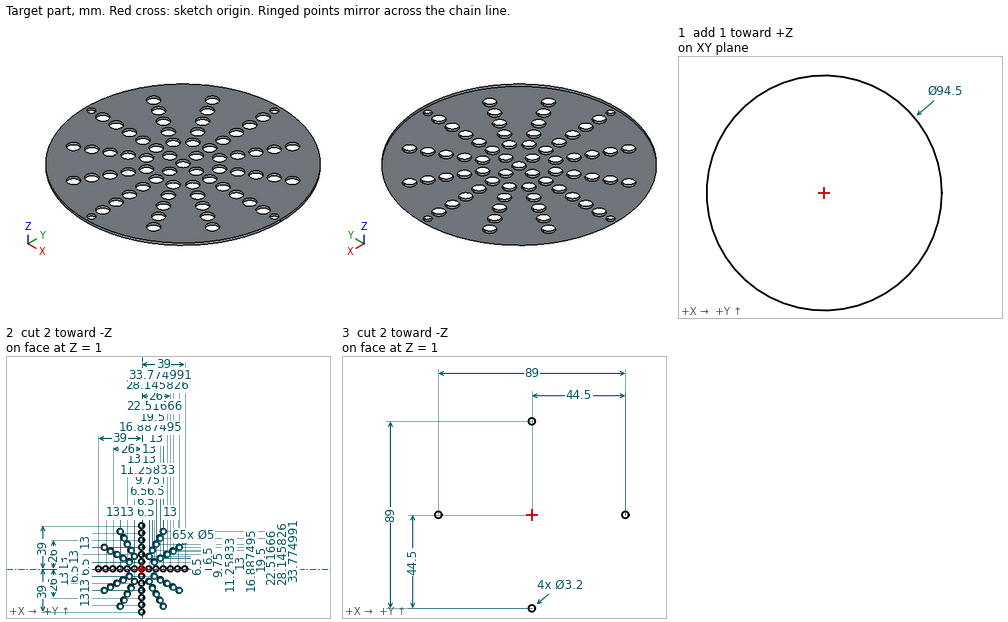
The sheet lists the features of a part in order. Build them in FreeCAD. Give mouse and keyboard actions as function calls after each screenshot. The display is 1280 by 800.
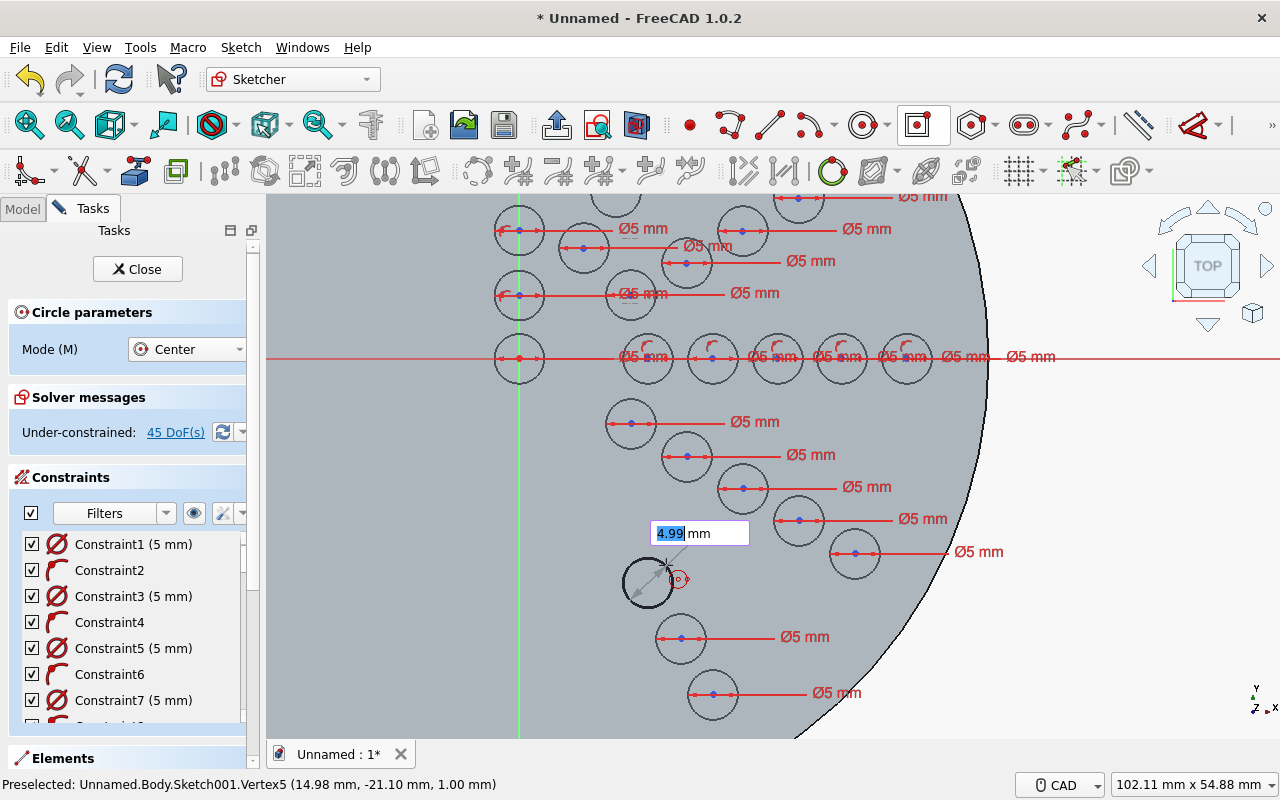
text(5)
key(Return)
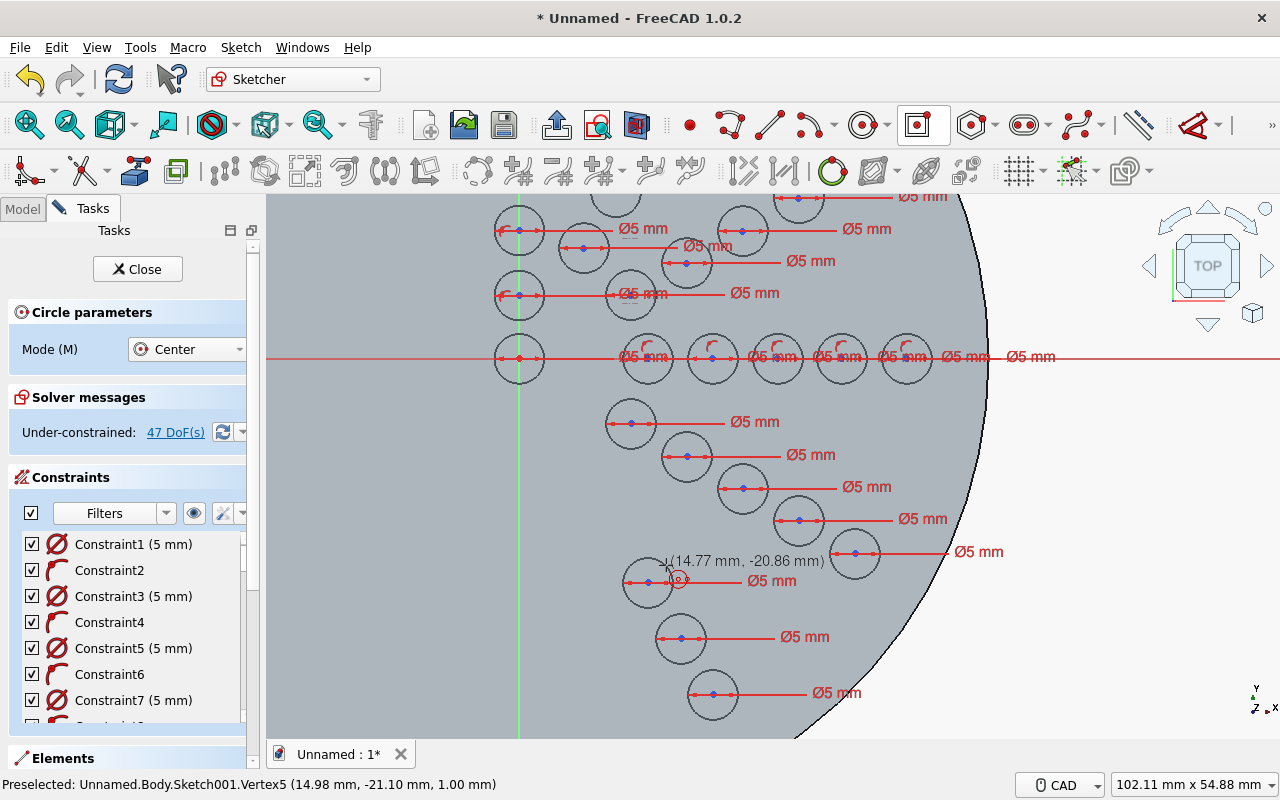
click(616, 527)
move(634, 509)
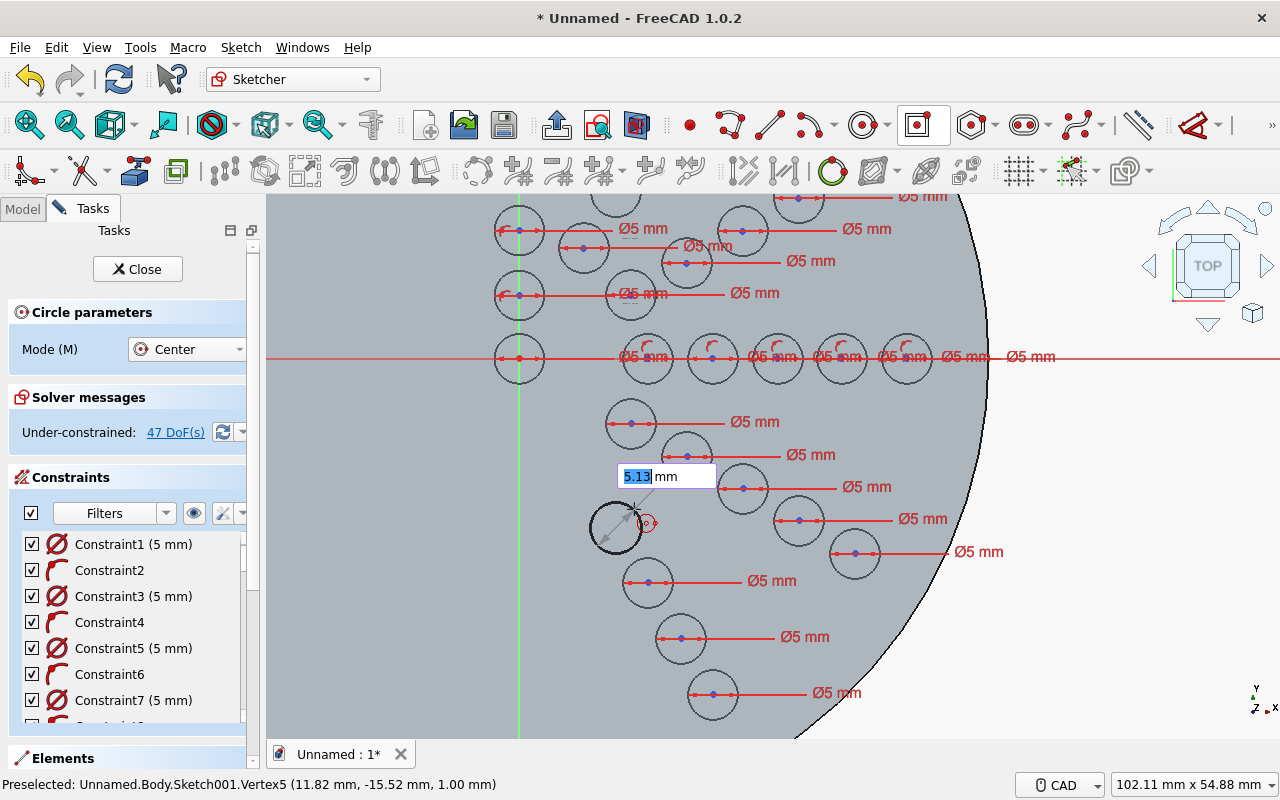
text(5)
key(Return)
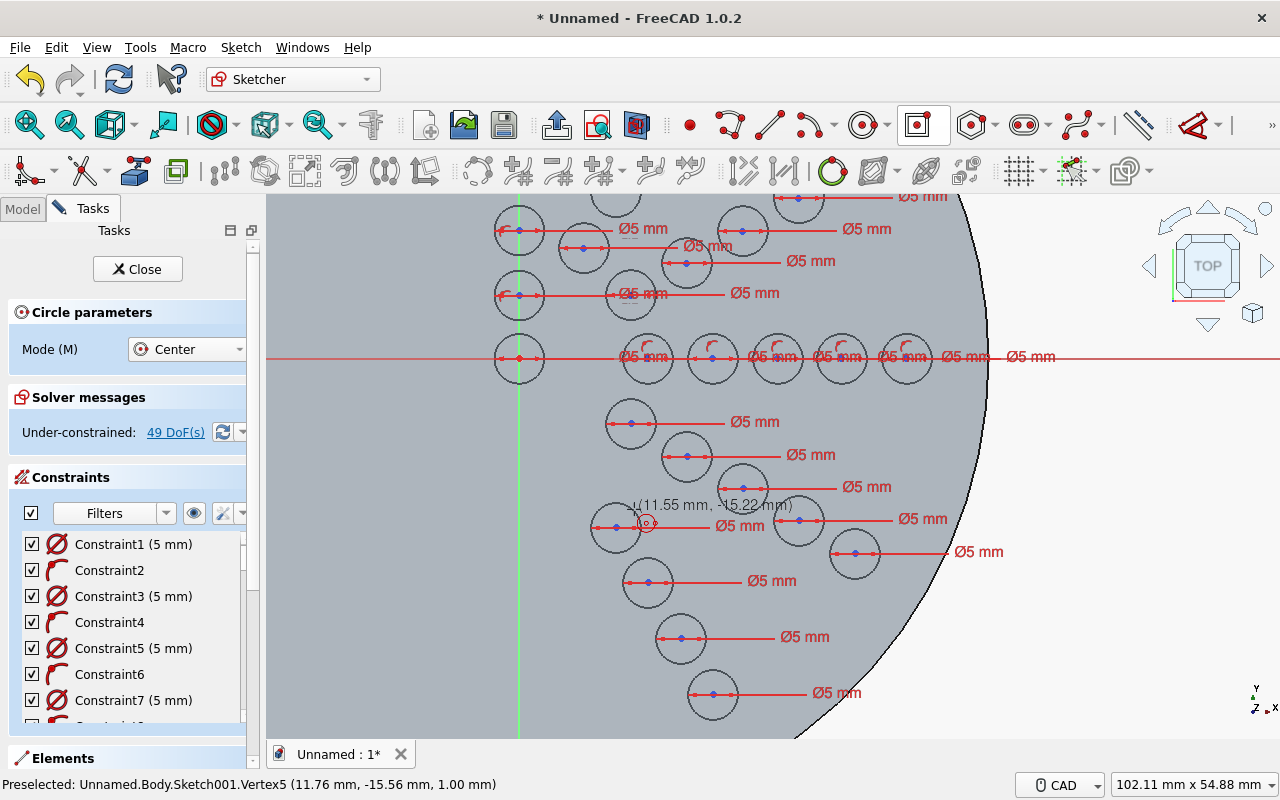
click(584, 471)
move(601, 453)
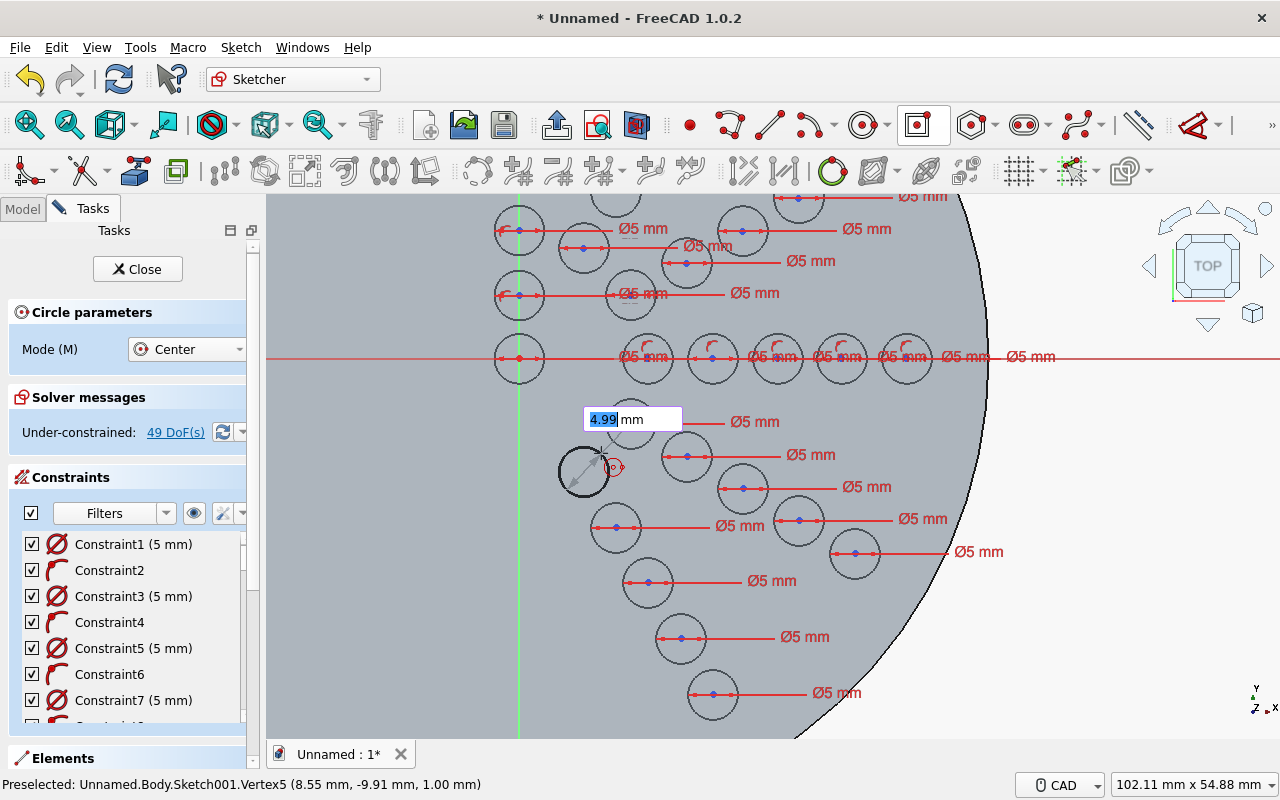
text(5)
key(Return)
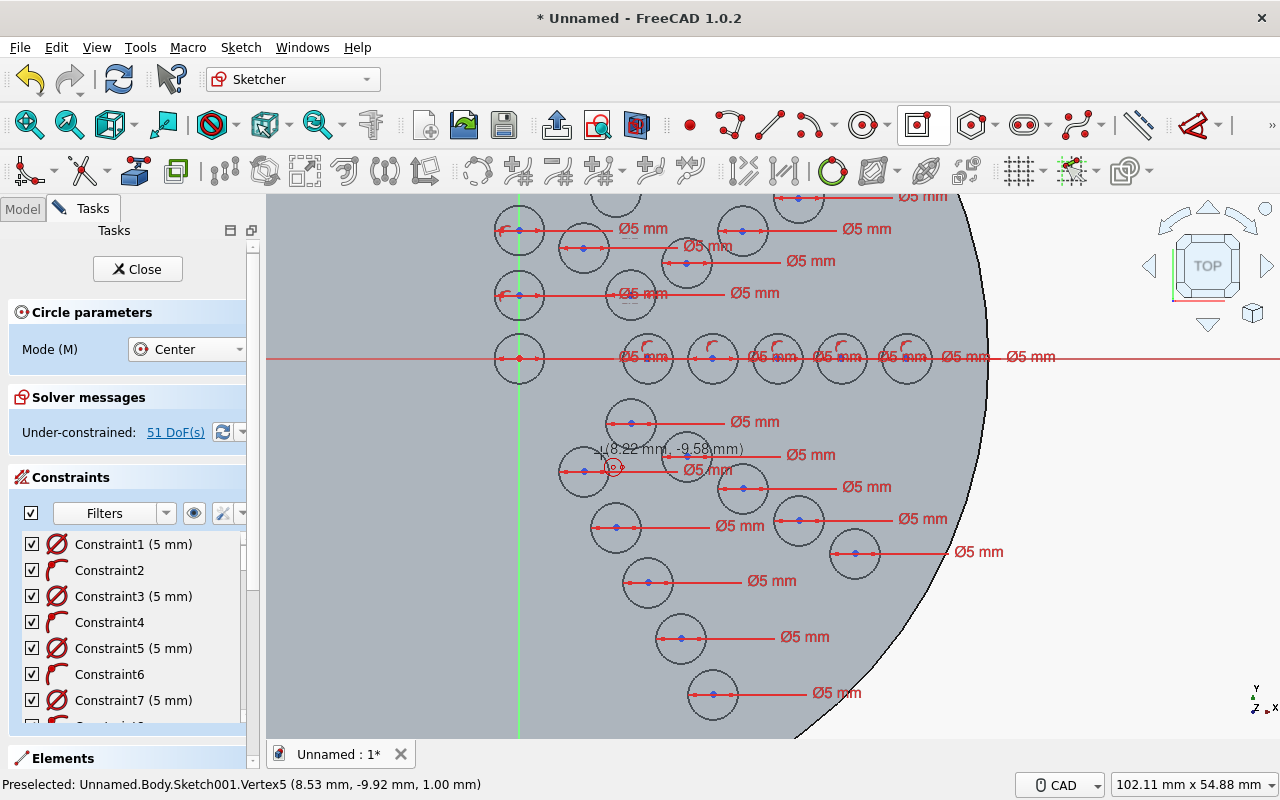
scroll(856, 554, down, 4)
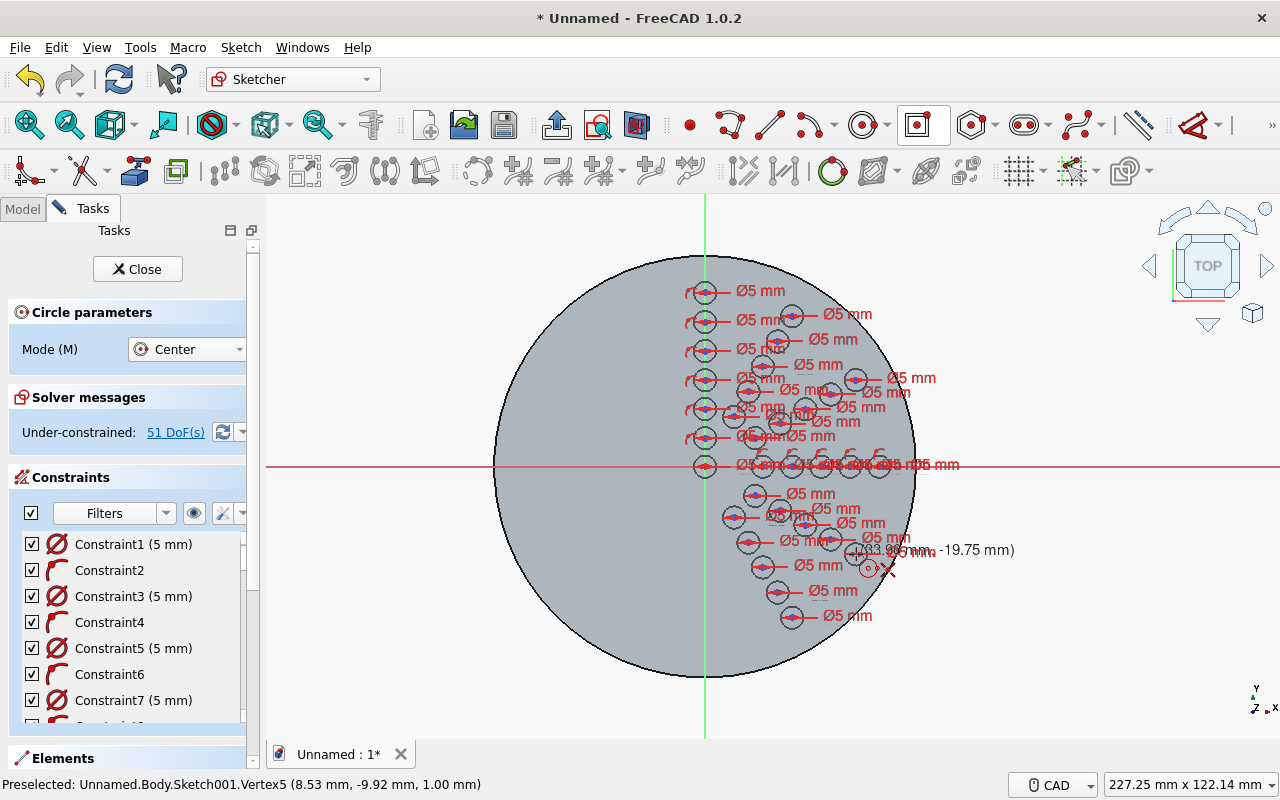
scroll(705, 641, up, 4)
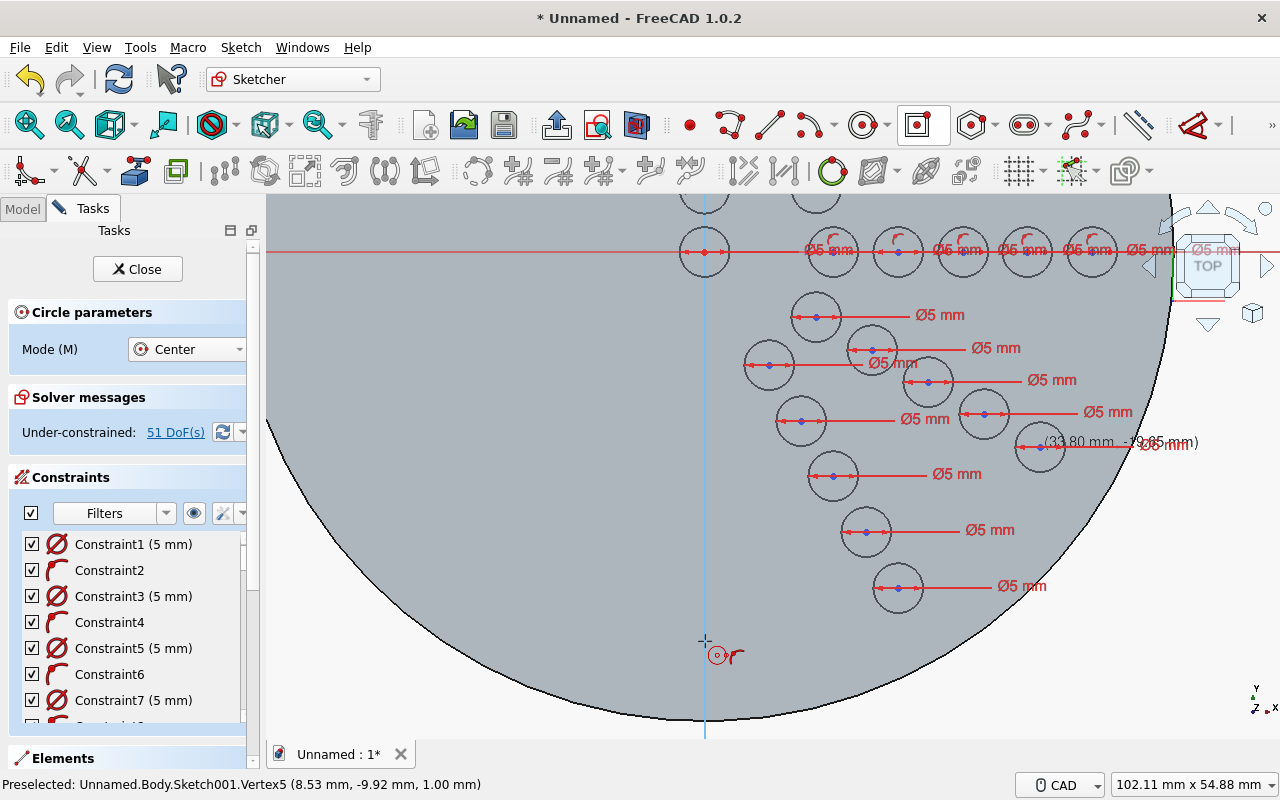
click(705, 639)
move(722, 622)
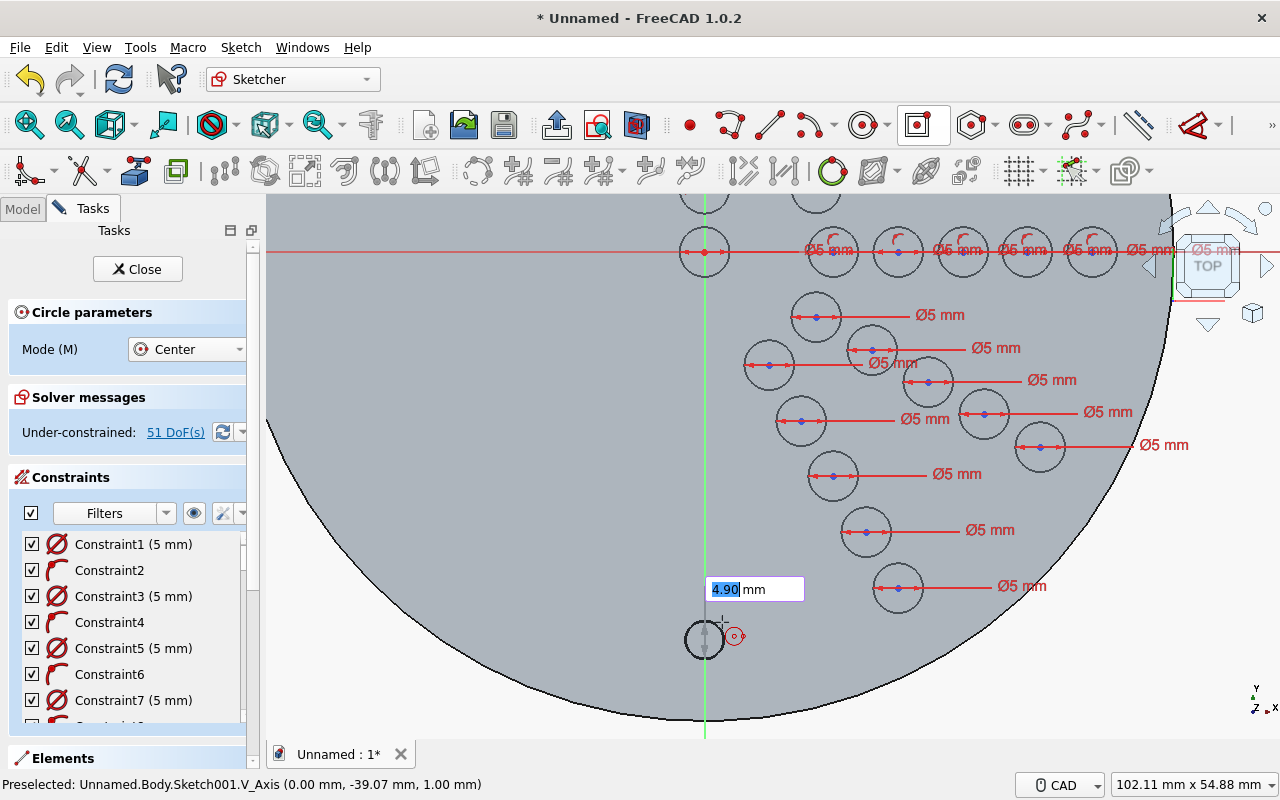
text(5)
key(Return)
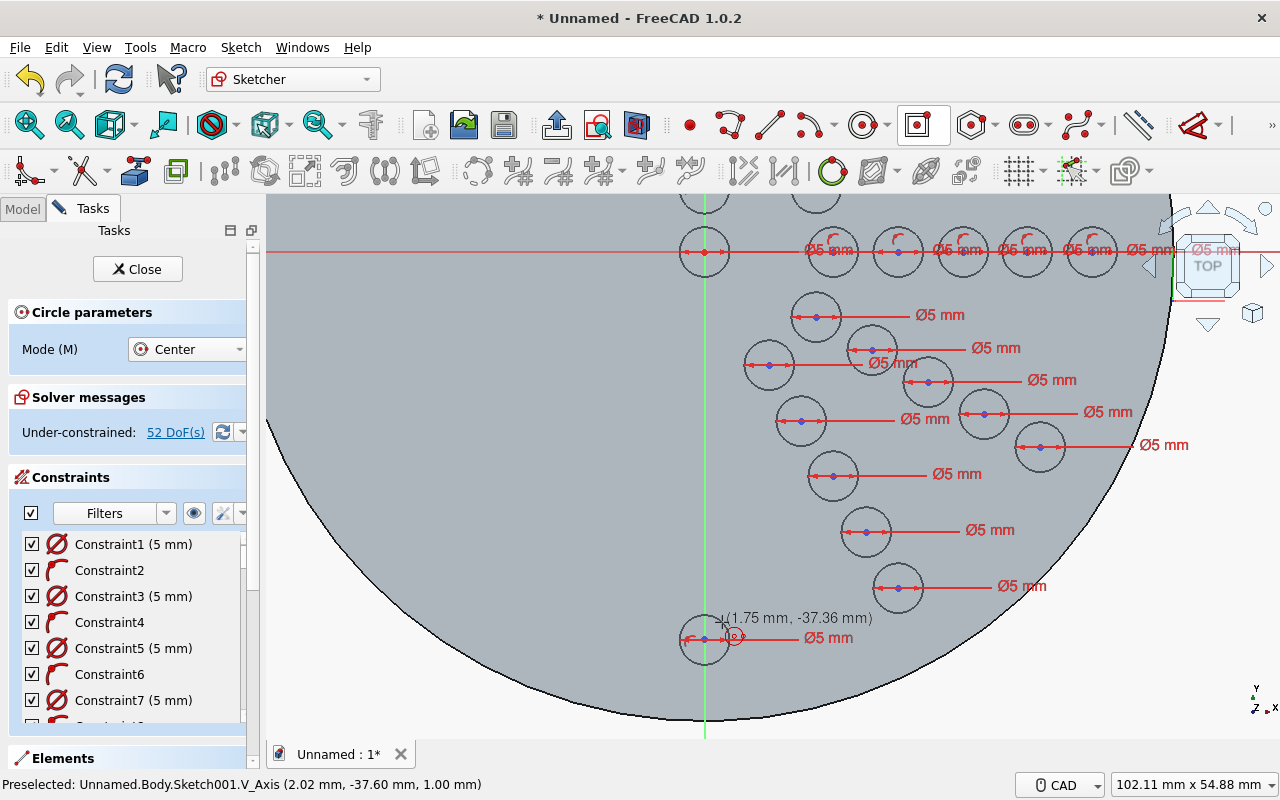
click(705, 575)
move(722, 557)